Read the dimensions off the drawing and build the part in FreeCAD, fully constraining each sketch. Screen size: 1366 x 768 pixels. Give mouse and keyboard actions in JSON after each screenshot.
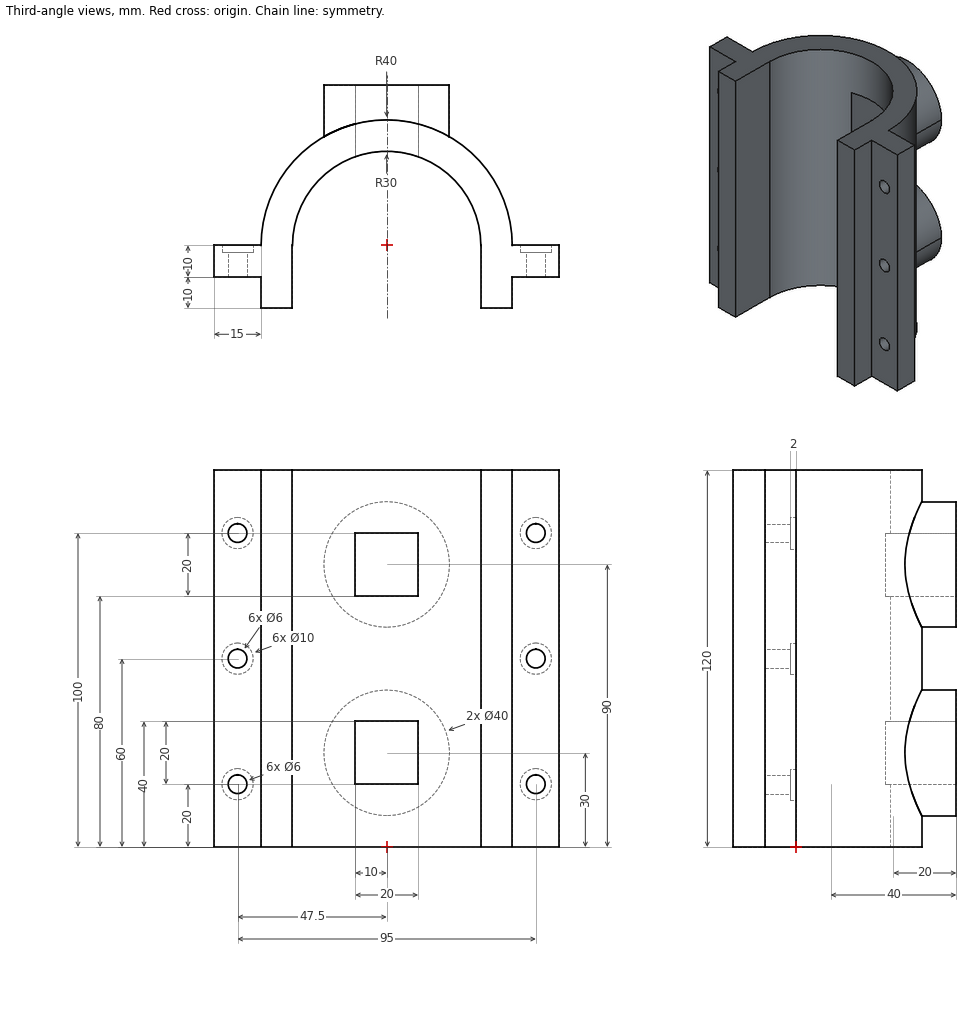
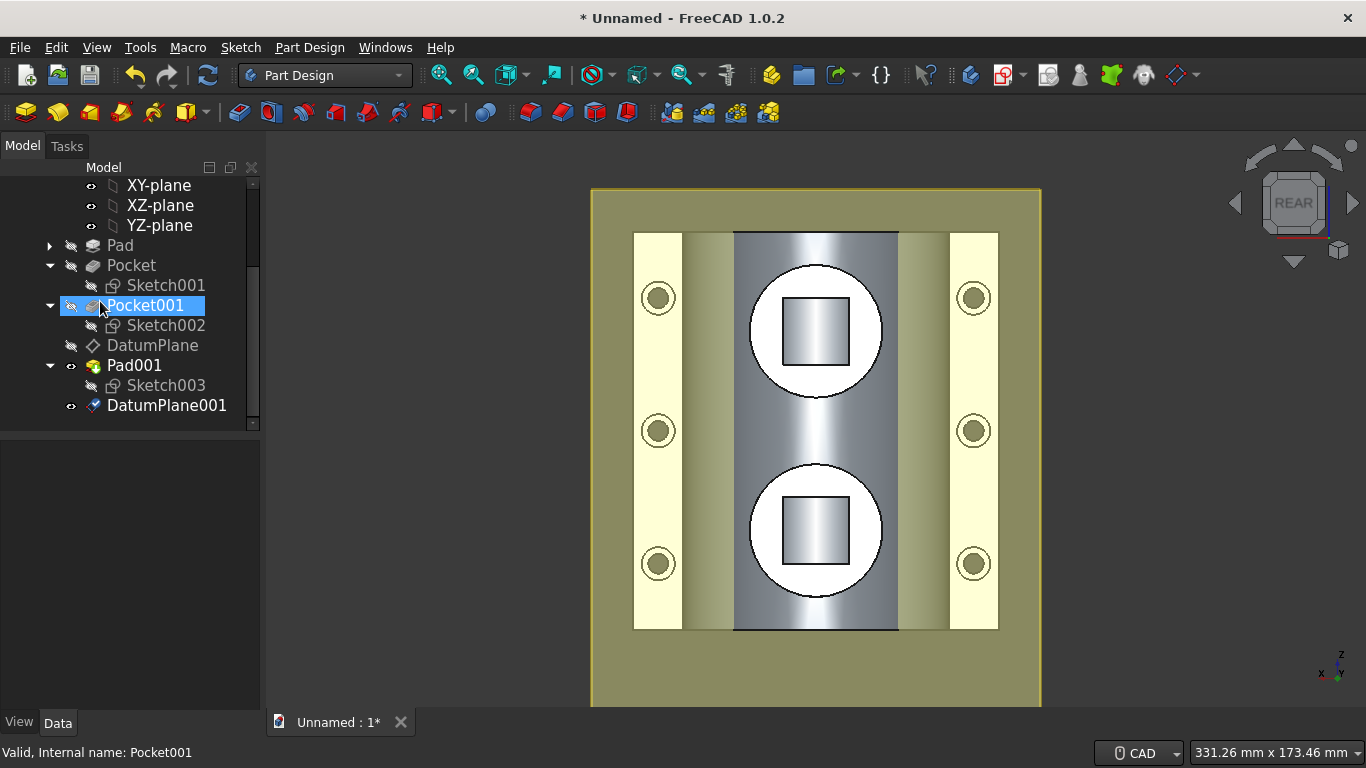
{"action": "left_click", "coordinate": [116, 406]}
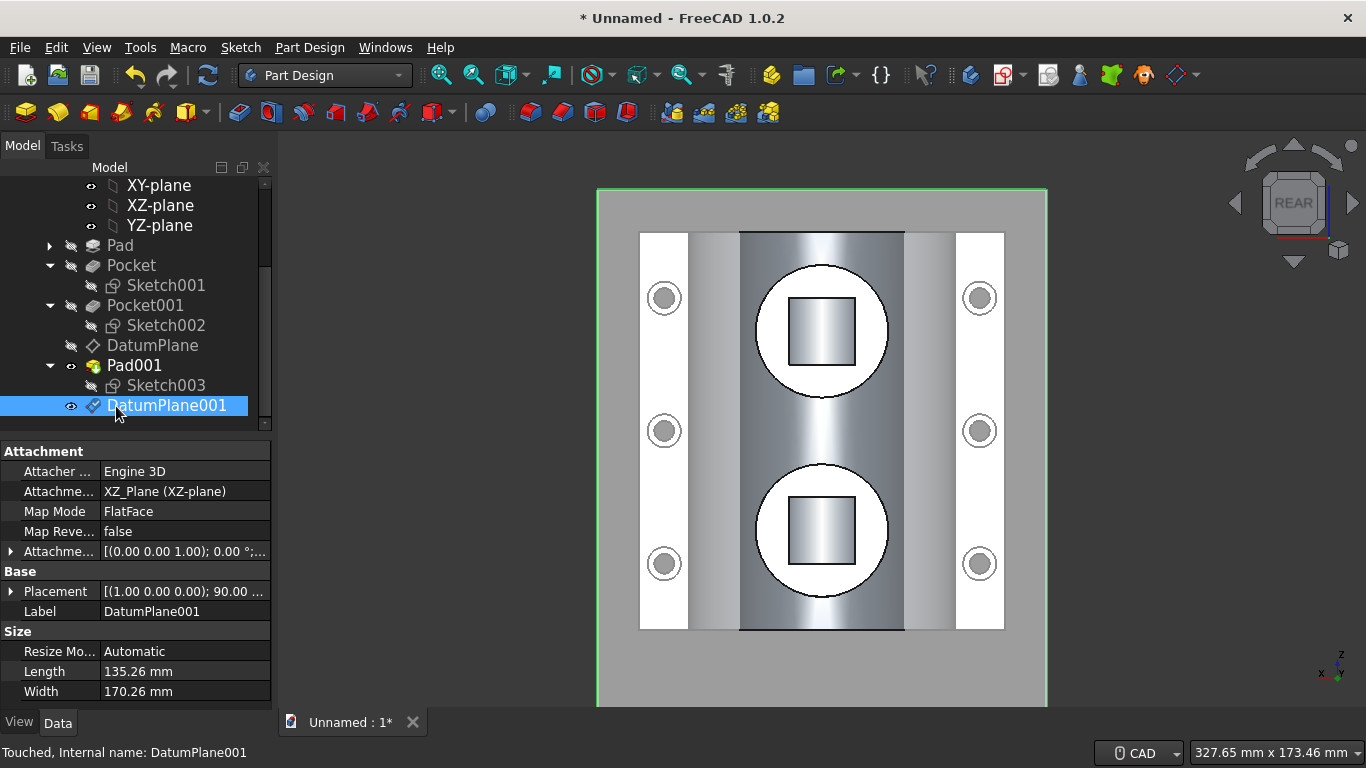
{"action": "left_click", "coordinate": [1004, 76]}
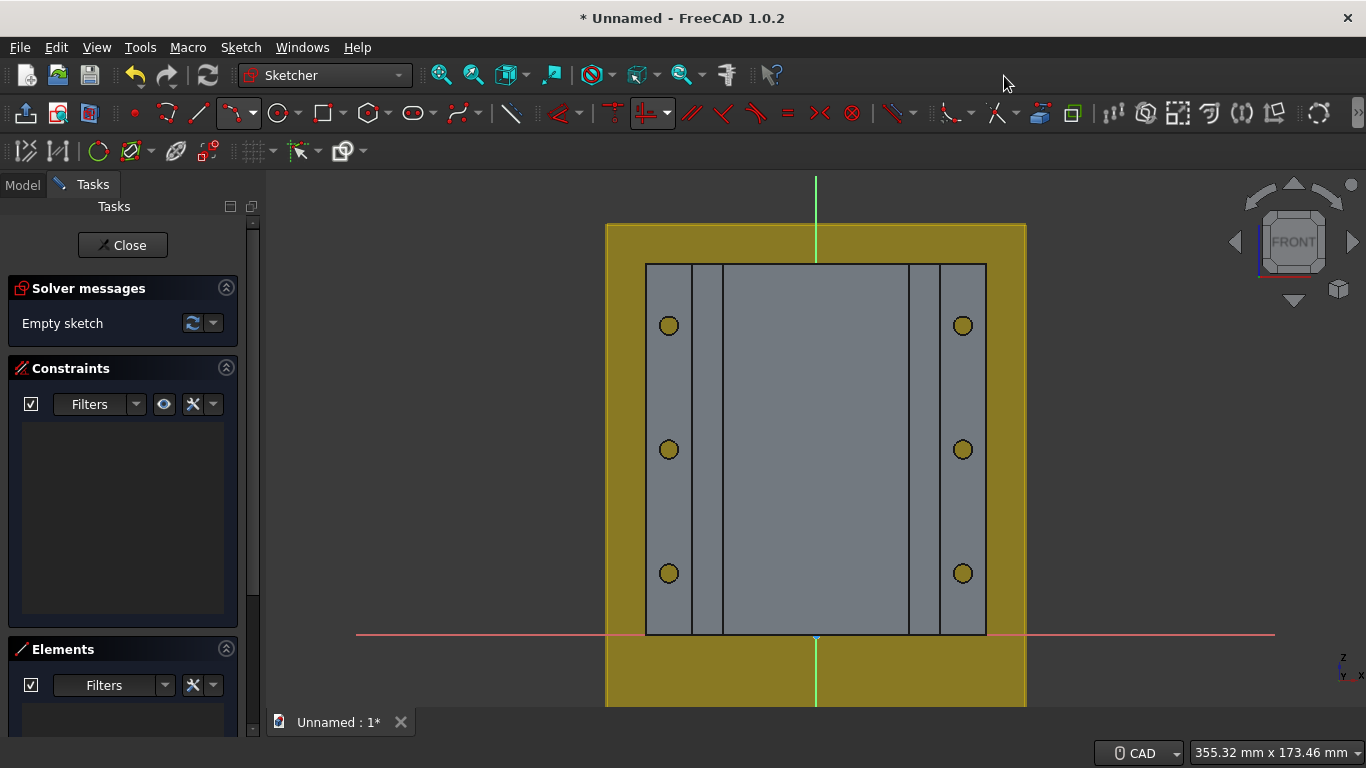
{"action": "left_click", "coordinate": [90, 114]}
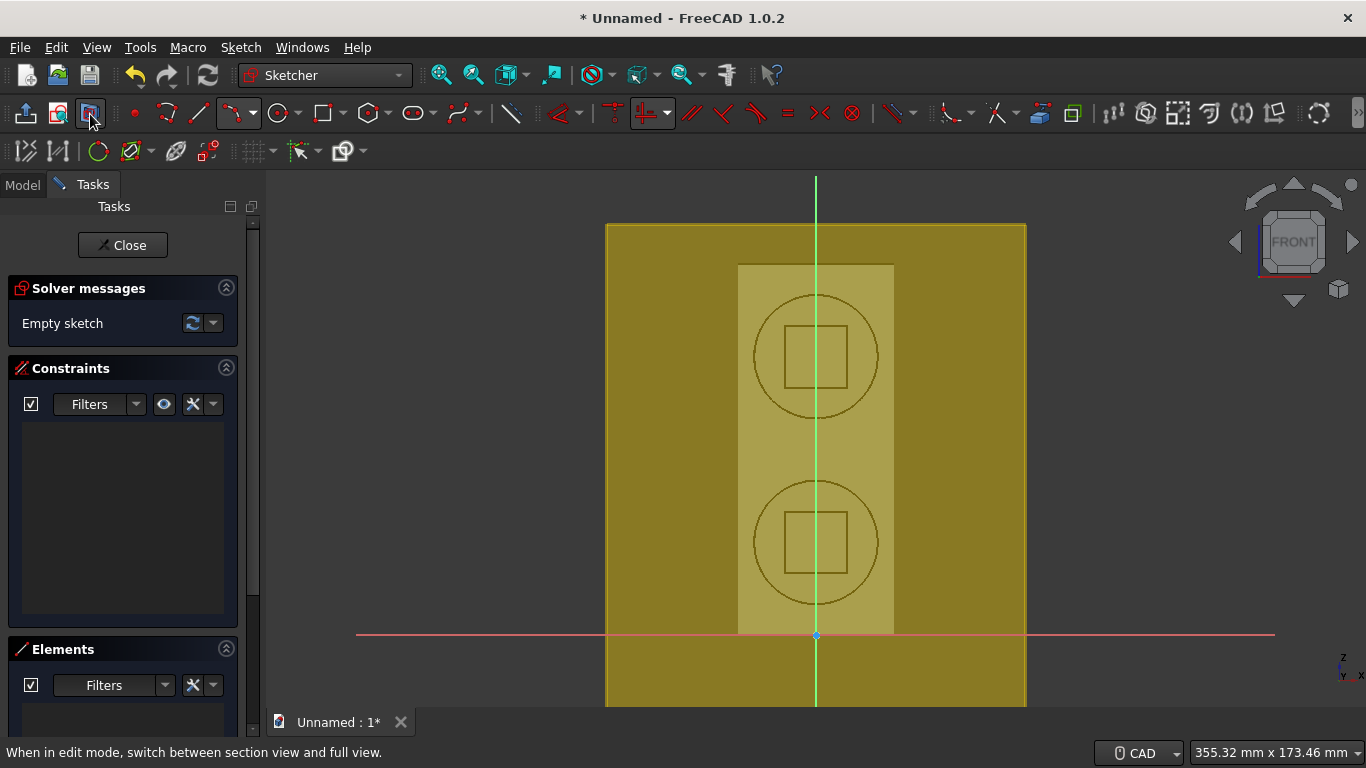
{"action": "left_click", "coordinate": [324, 114]}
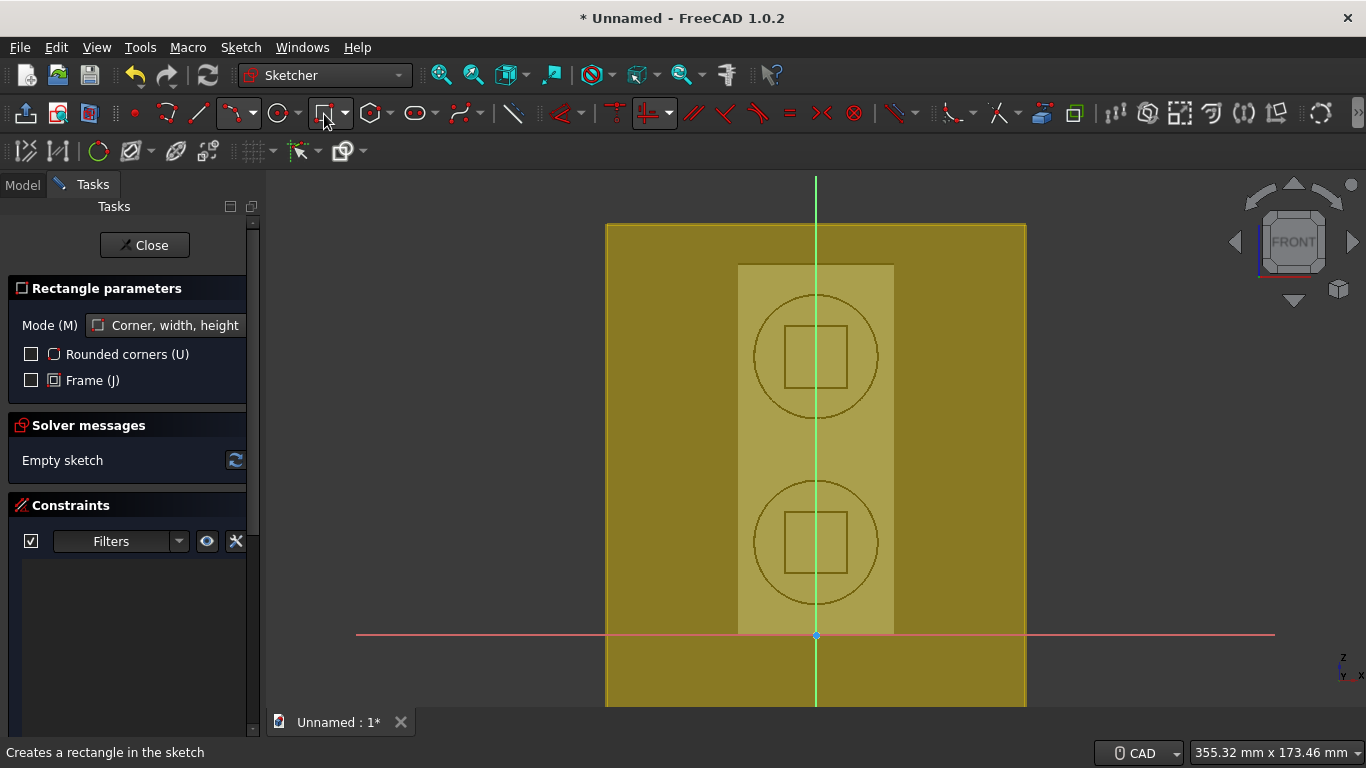
{"action": "left_click", "coordinate": [785, 512]}
{"action": "left_click", "coordinate": [847, 573]}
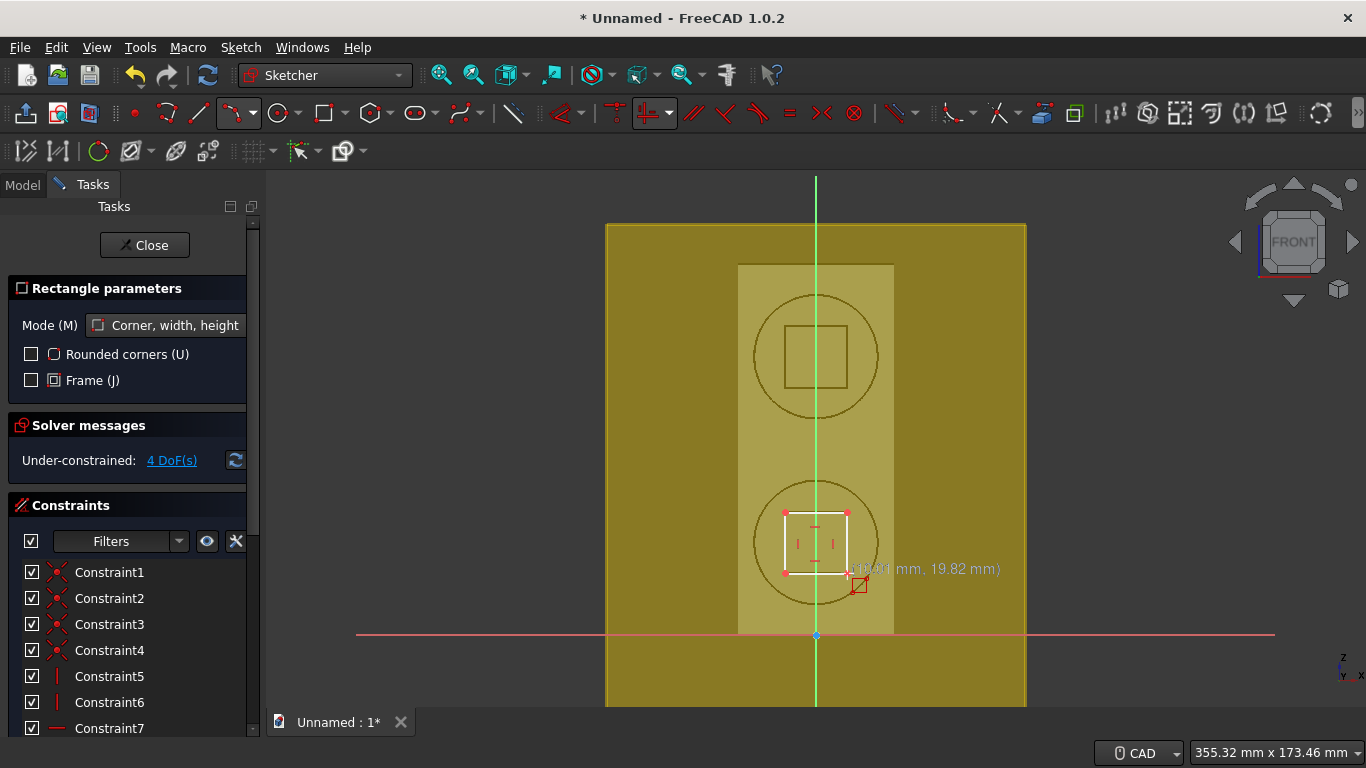
{"action": "left_click", "coordinate": [785, 326]}
{"action": "left_click", "coordinate": [847, 388]}
{"action": "key", "text": "Escape"}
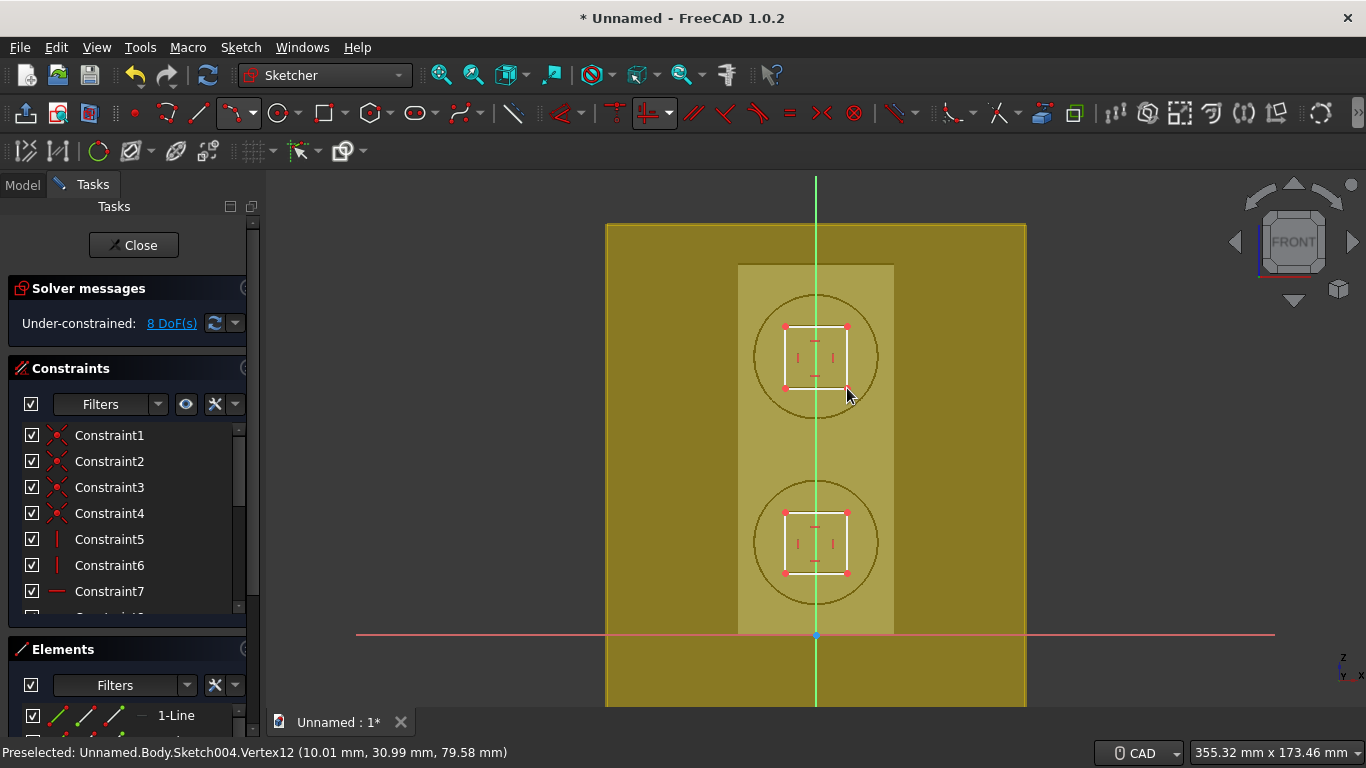
{"action": "left_click", "coordinate": [785, 531]}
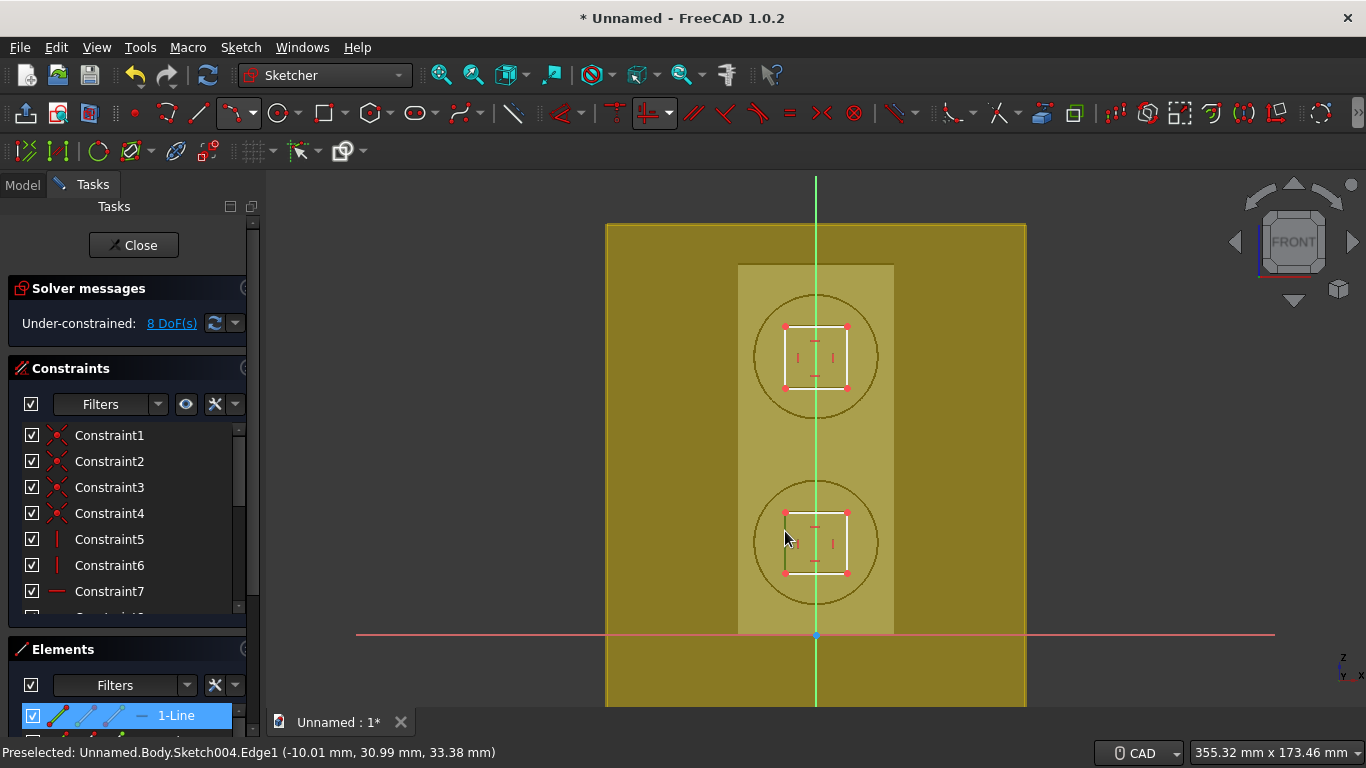
{"action": "left_click", "coordinate": [584, 114]}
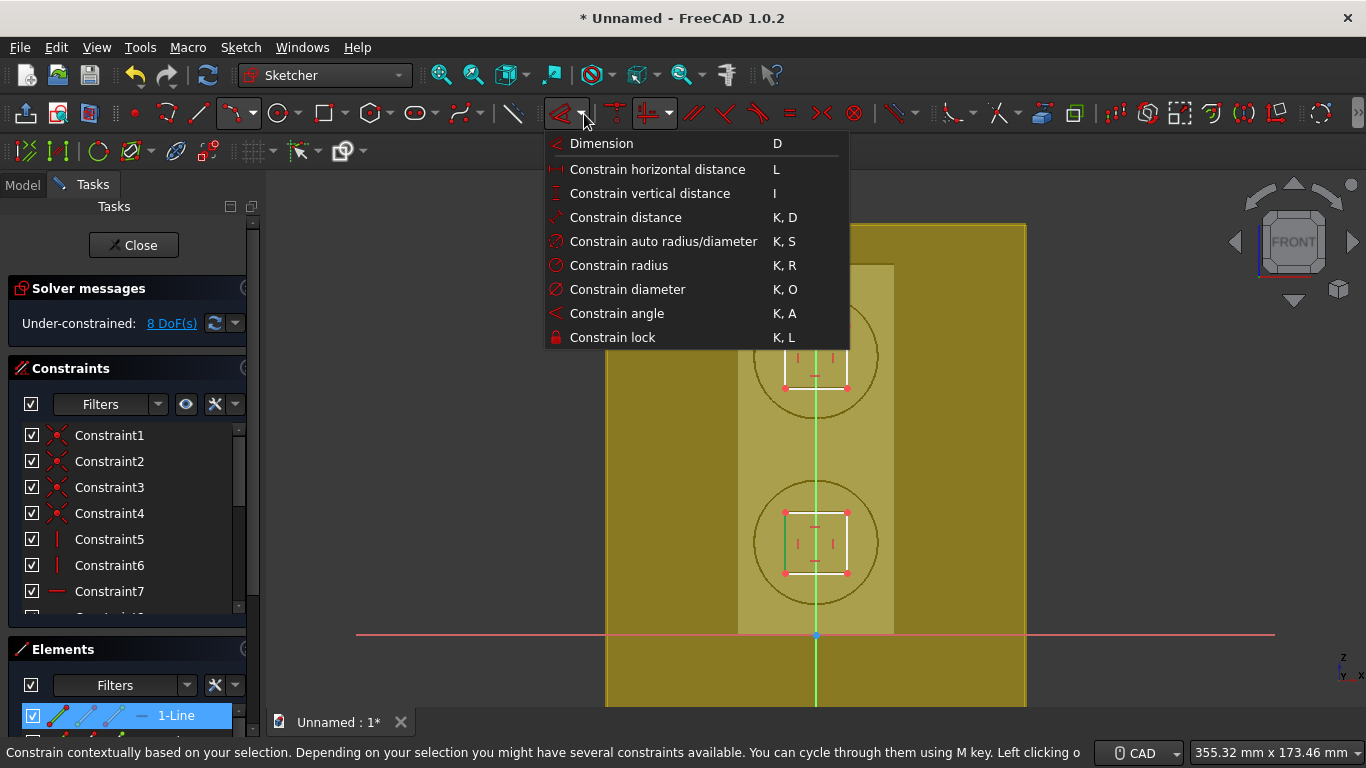
{"action": "left_click", "coordinate": [697, 193]}